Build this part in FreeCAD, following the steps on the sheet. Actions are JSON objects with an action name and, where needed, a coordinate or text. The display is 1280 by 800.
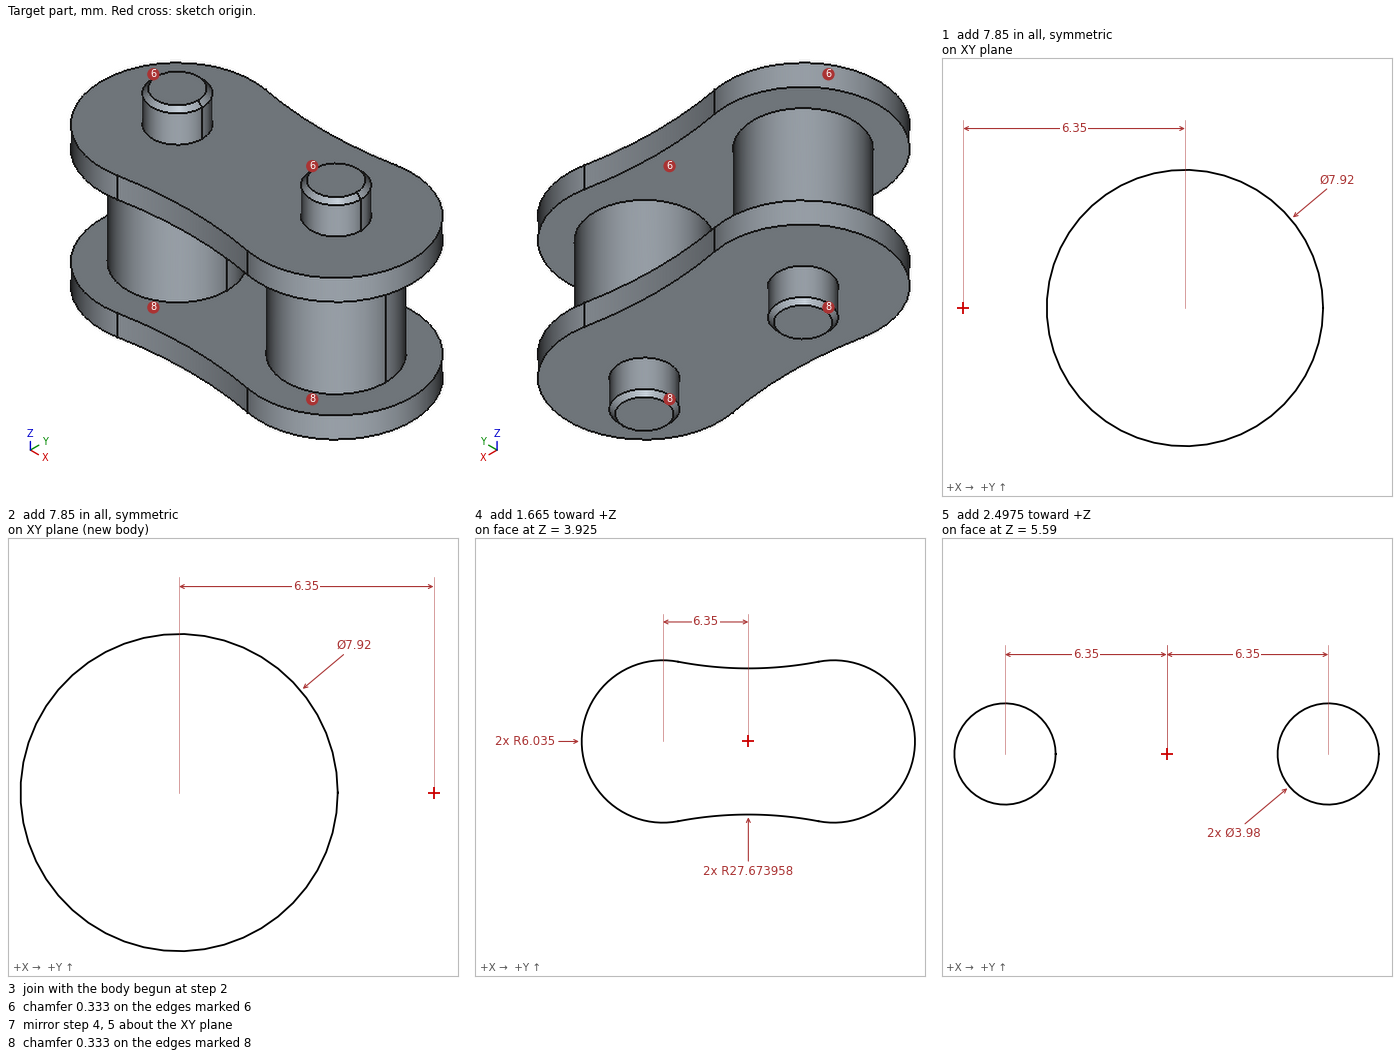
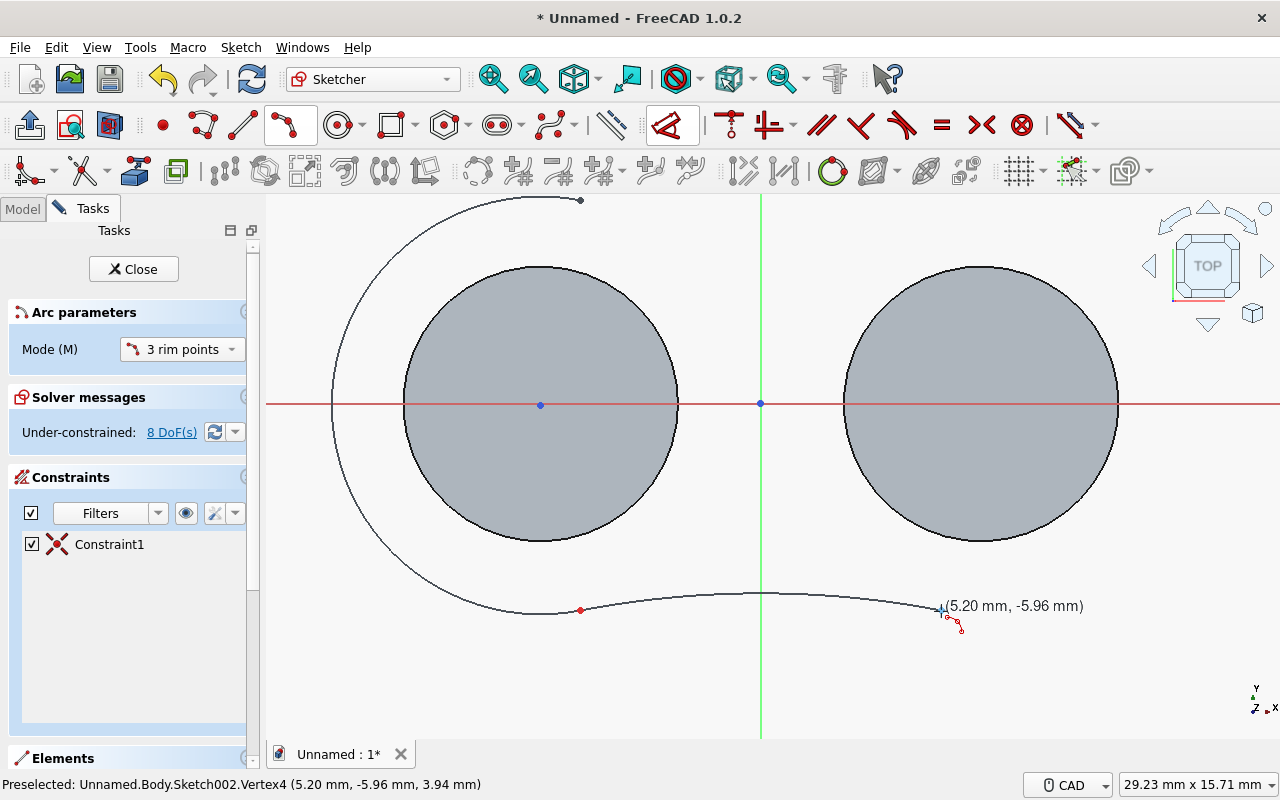
{"action": "scroll", "coordinate": [590, 594], "scroll_direction": "down", "scroll_amount": 2}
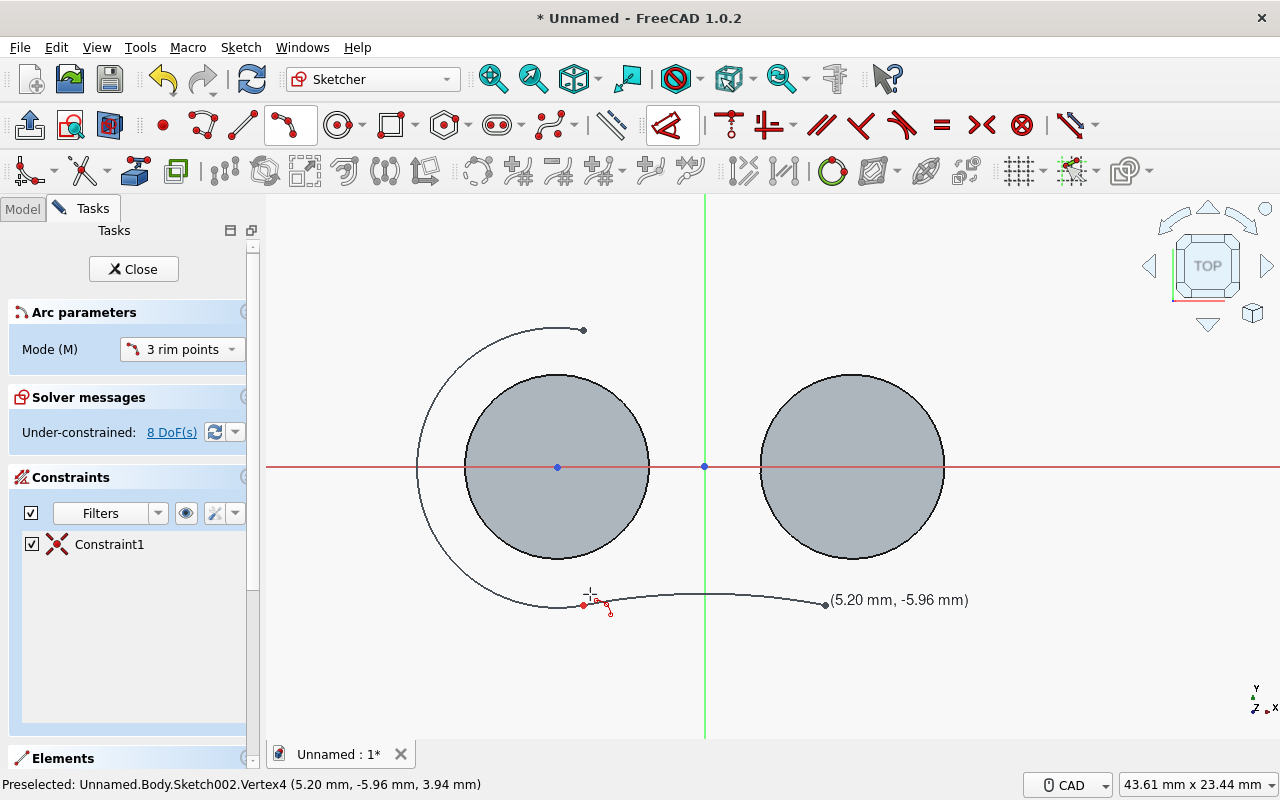
{"action": "left_click", "coordinate": [826, 329]}
{"action": "left_click", "coordinate": [984, 515]}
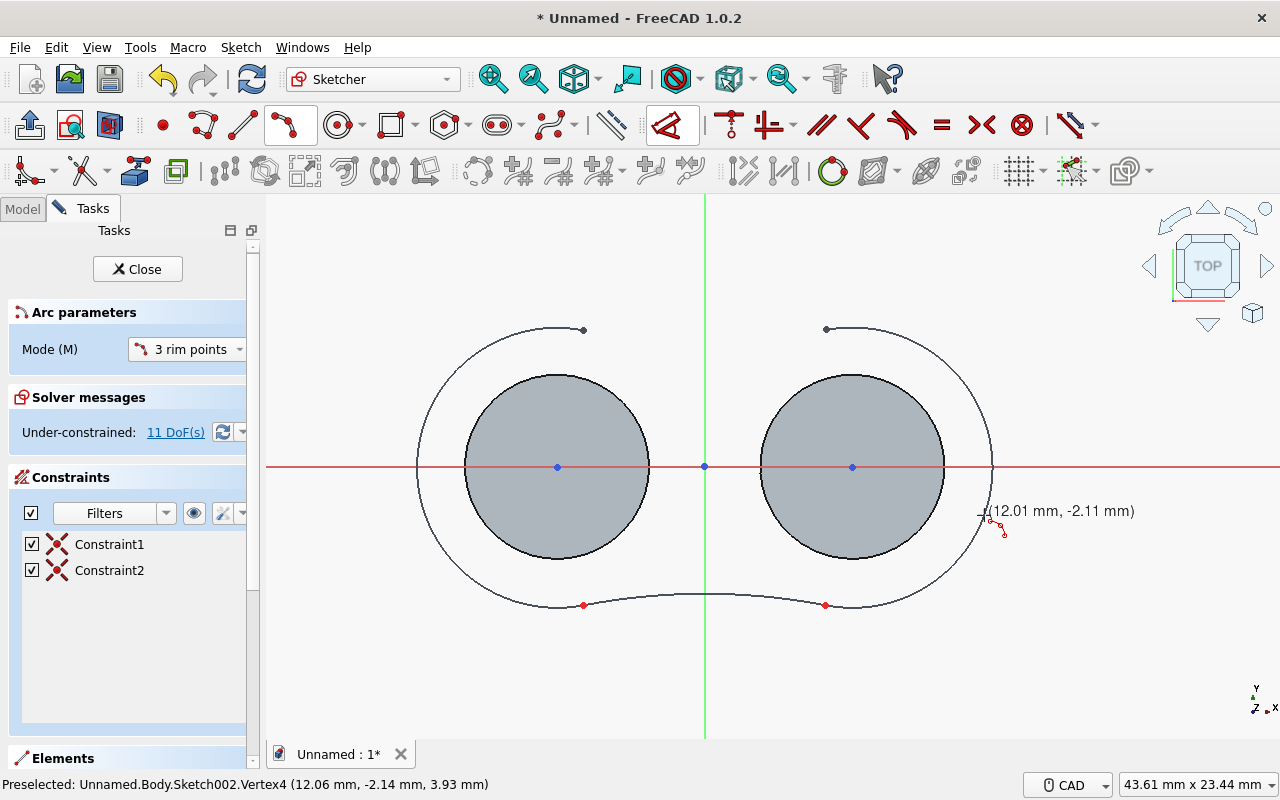
{"action": "left_click", "coordinate": [826, 330]}
{"action": "left_click", "coordinate": [584, 330]}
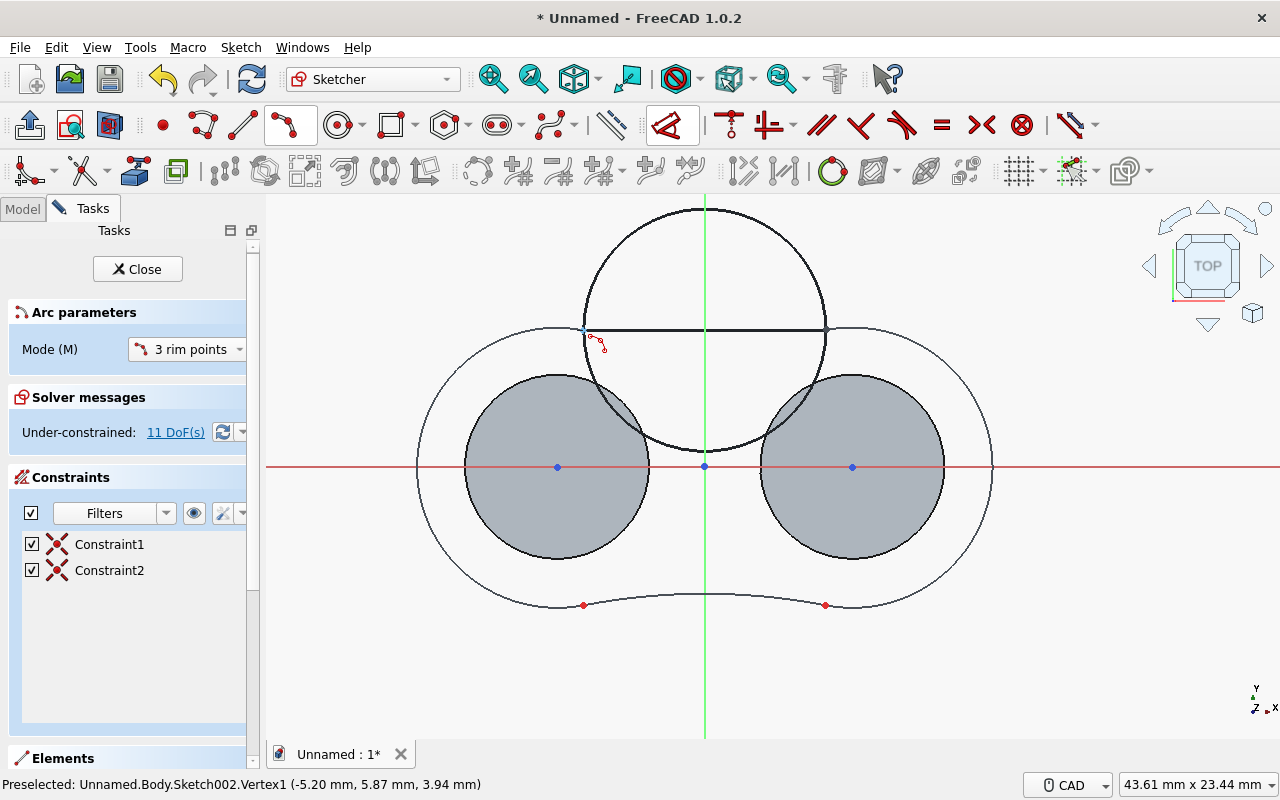
{"action": "scroll", "coordinate": [680, 340], "scroll_direction": "up", "scroll_amount": 2}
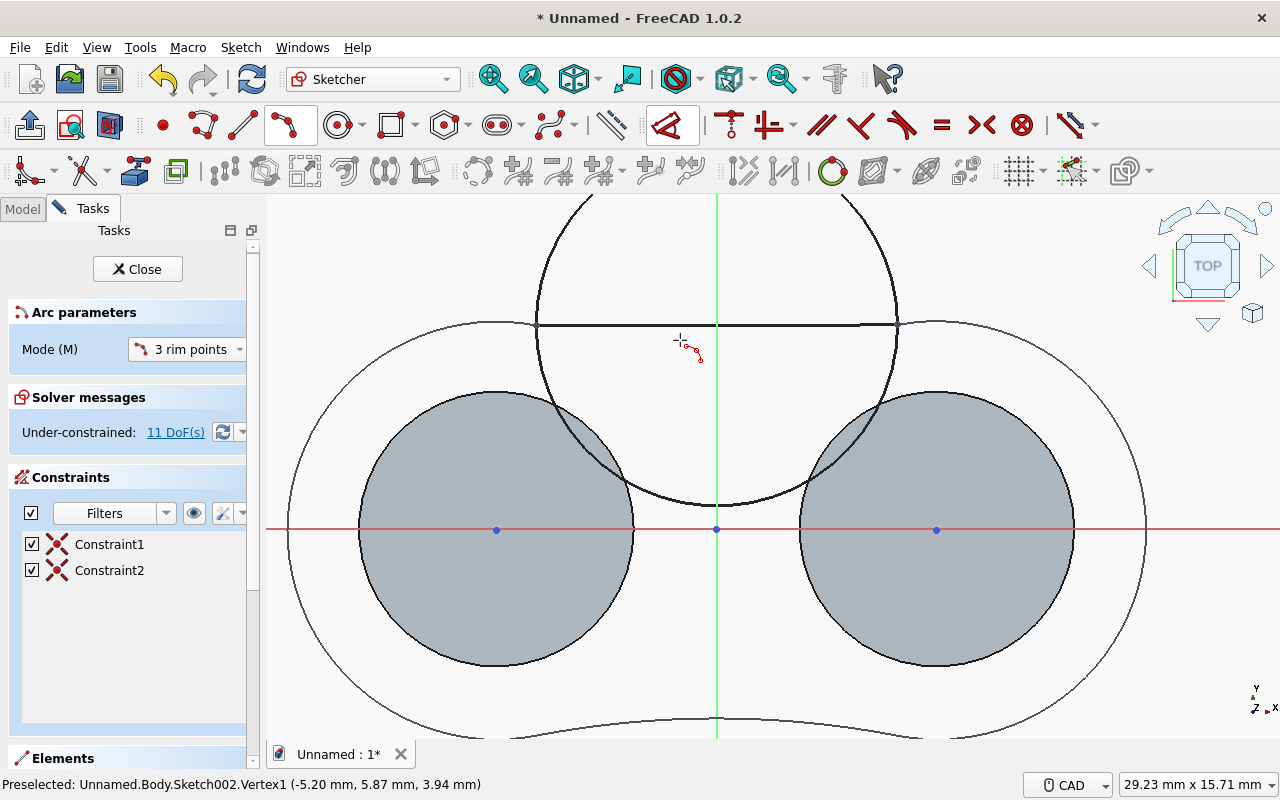
{"action": "left_click", "coordinate": [680, 340]}
{"action": "key", "text": "Escape"}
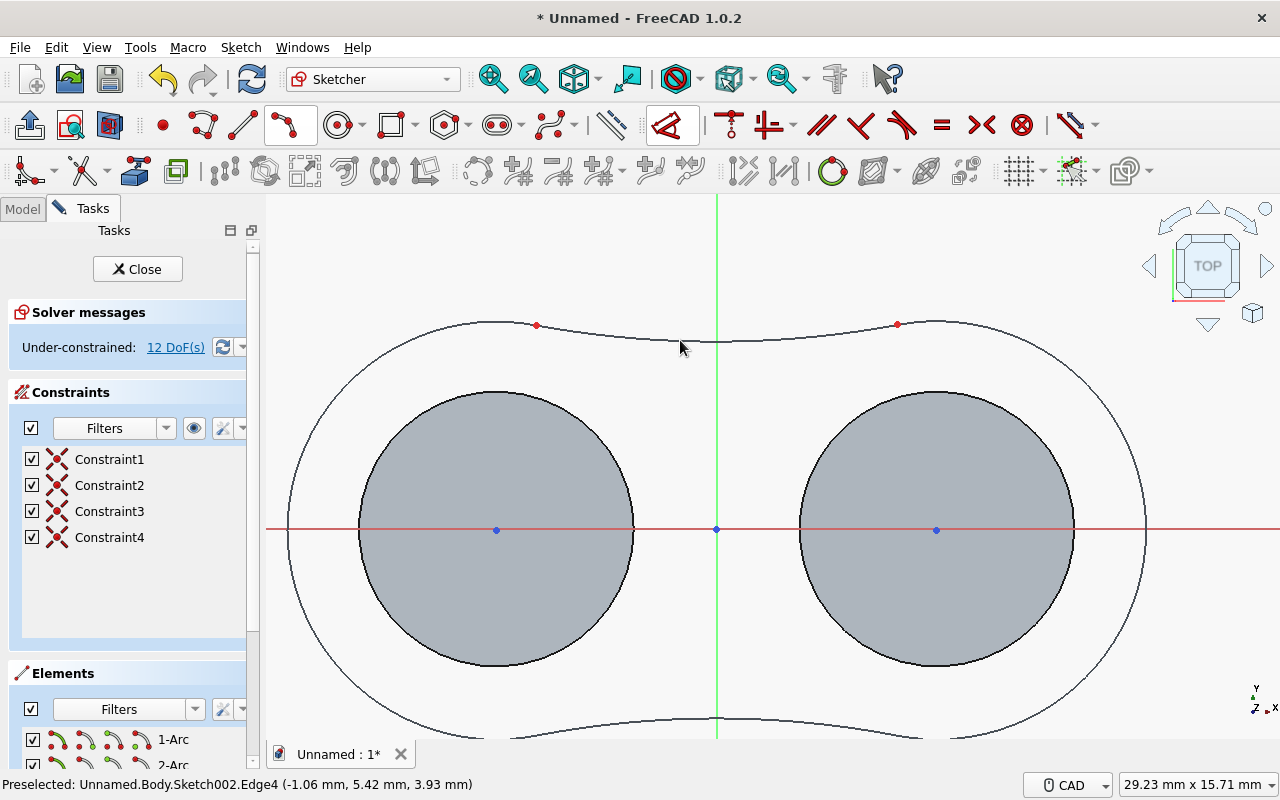
{"action": "left_click", "coordinate": [337, 395]}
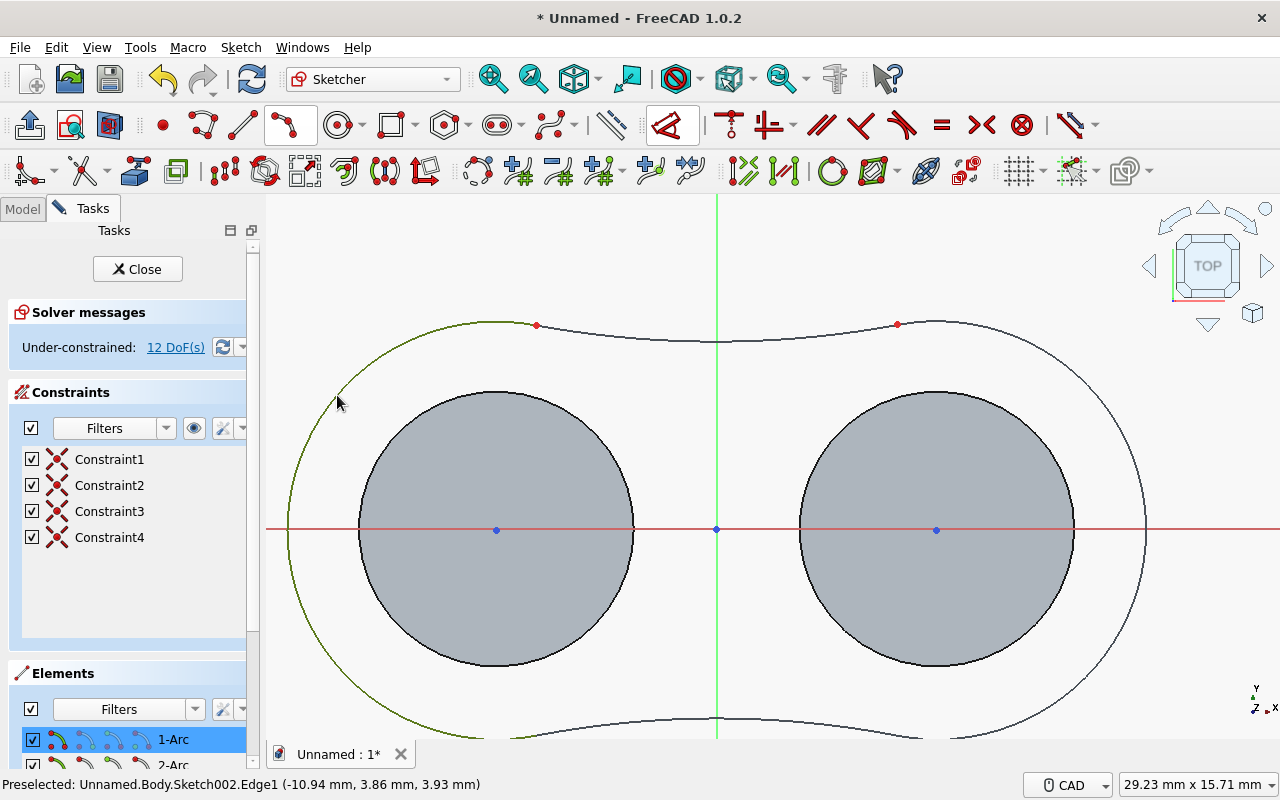
{"action": "scroll", "coordinate": [680, 339], "scroll_direction": "down", "scroll_amount": 2}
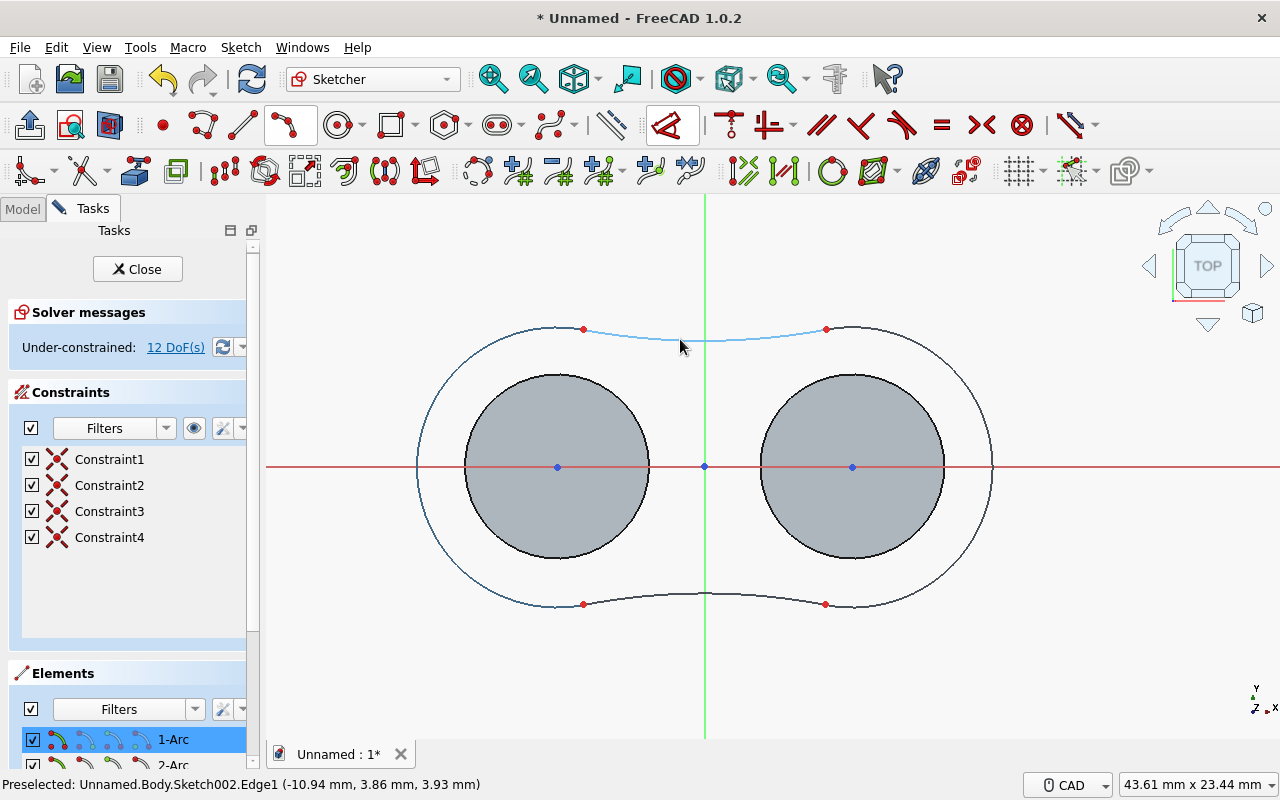
{"action": "left_click", "coordinate": [753, 595]}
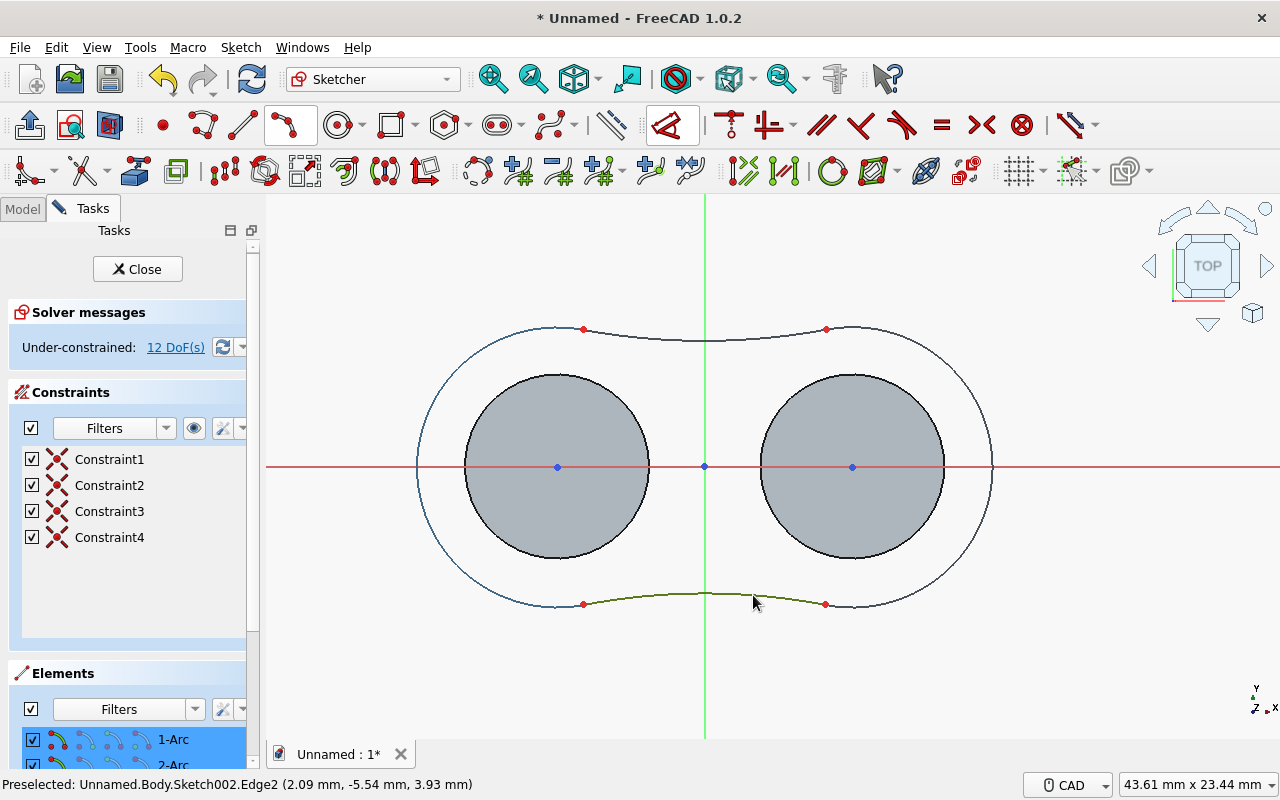
{"action": "left_click", "coordinate": [902, 126]}